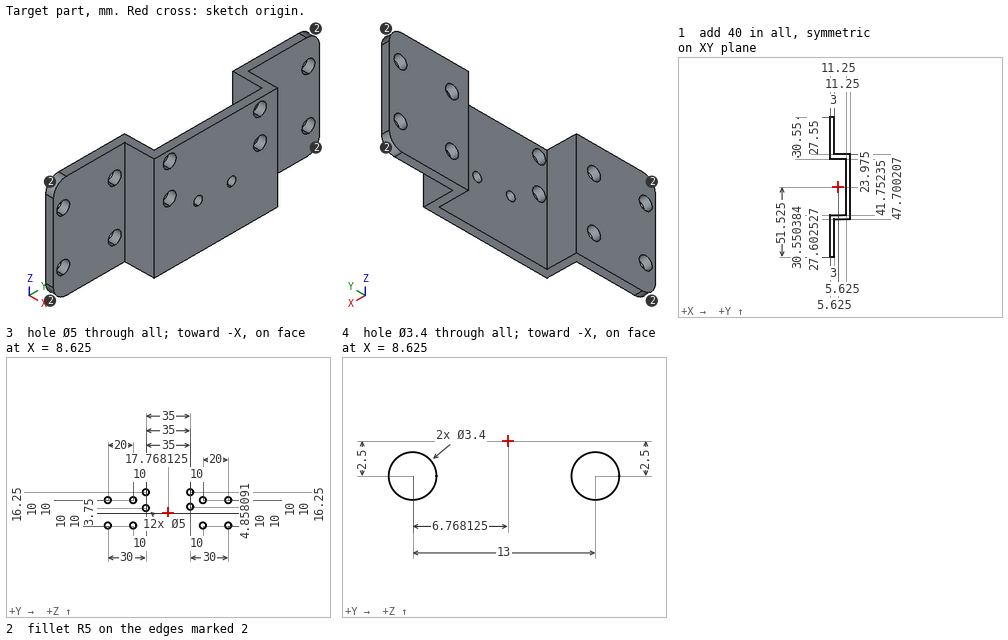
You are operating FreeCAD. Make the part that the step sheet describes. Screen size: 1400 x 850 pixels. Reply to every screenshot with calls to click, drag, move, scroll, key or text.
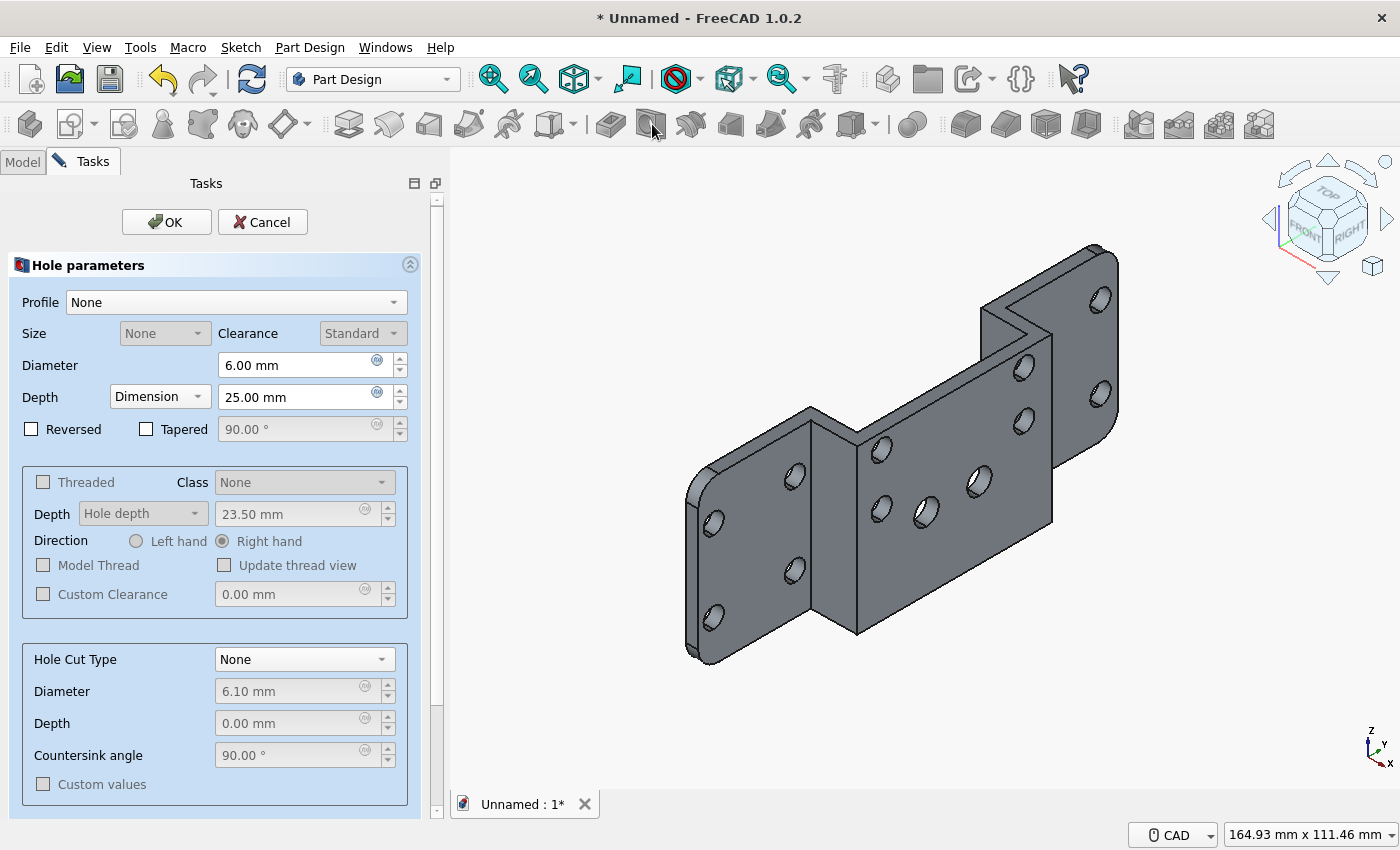
triple_click(305, 365)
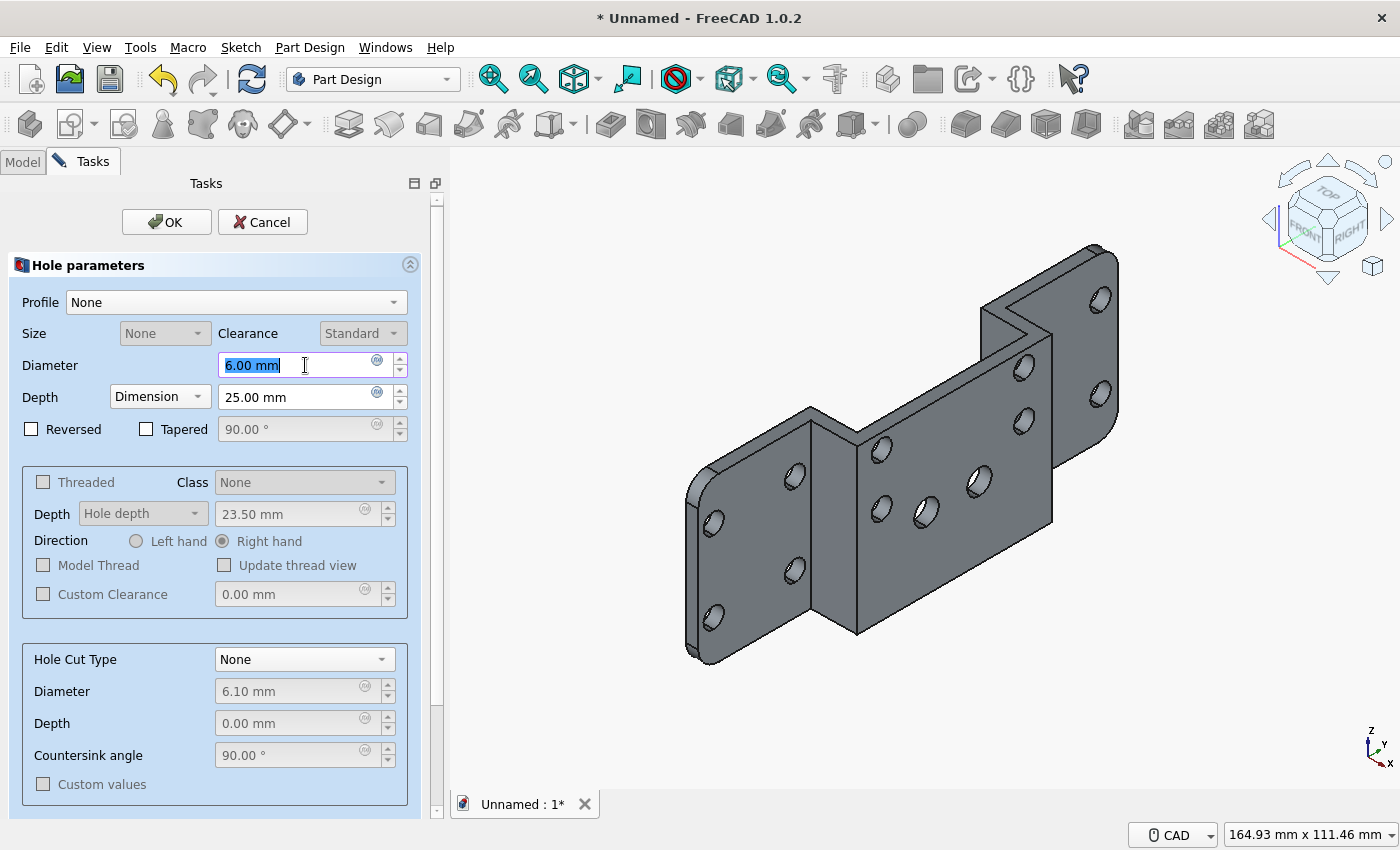
text(3.4)
key(Tab)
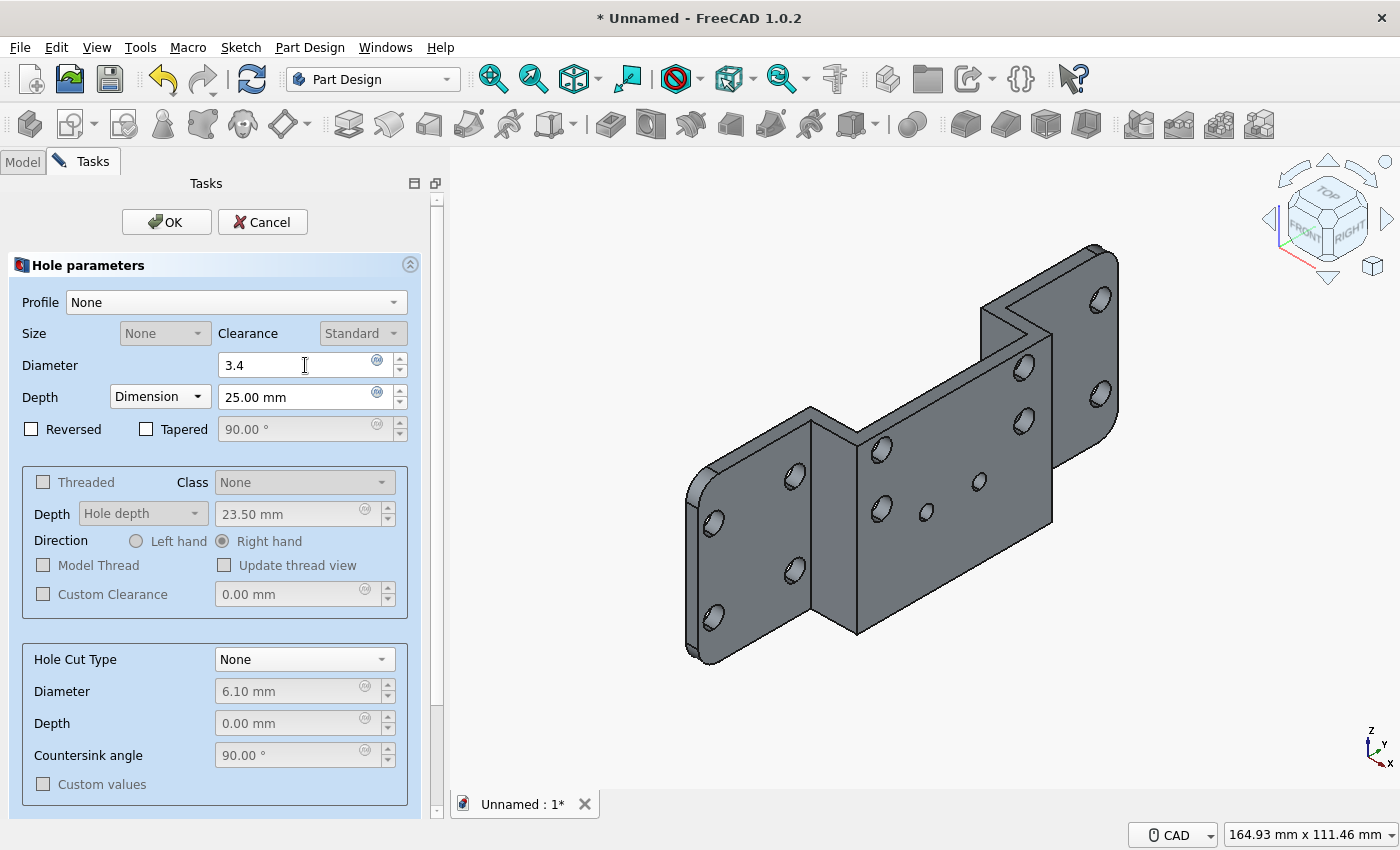
click(161, 396)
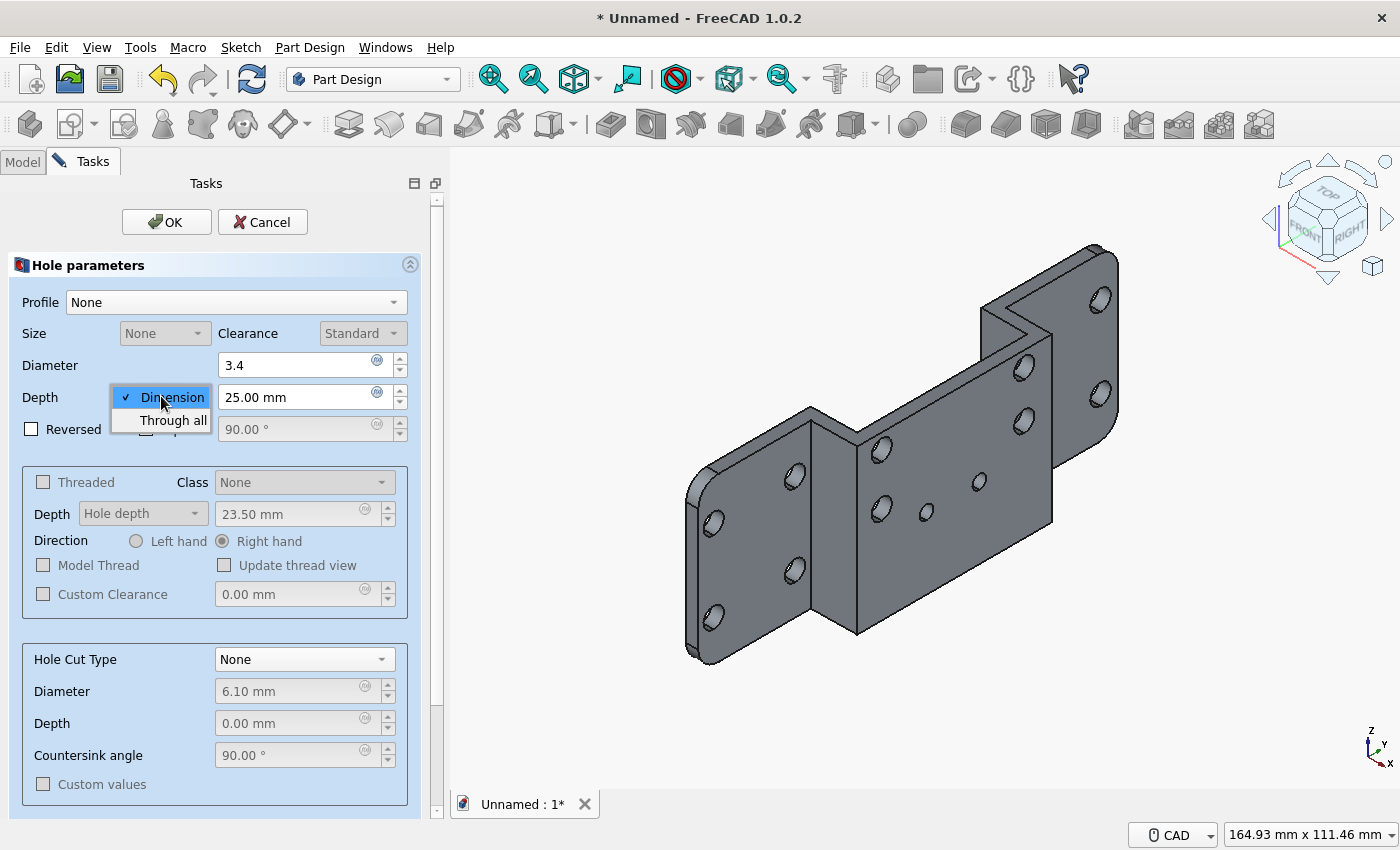
click(160, 420)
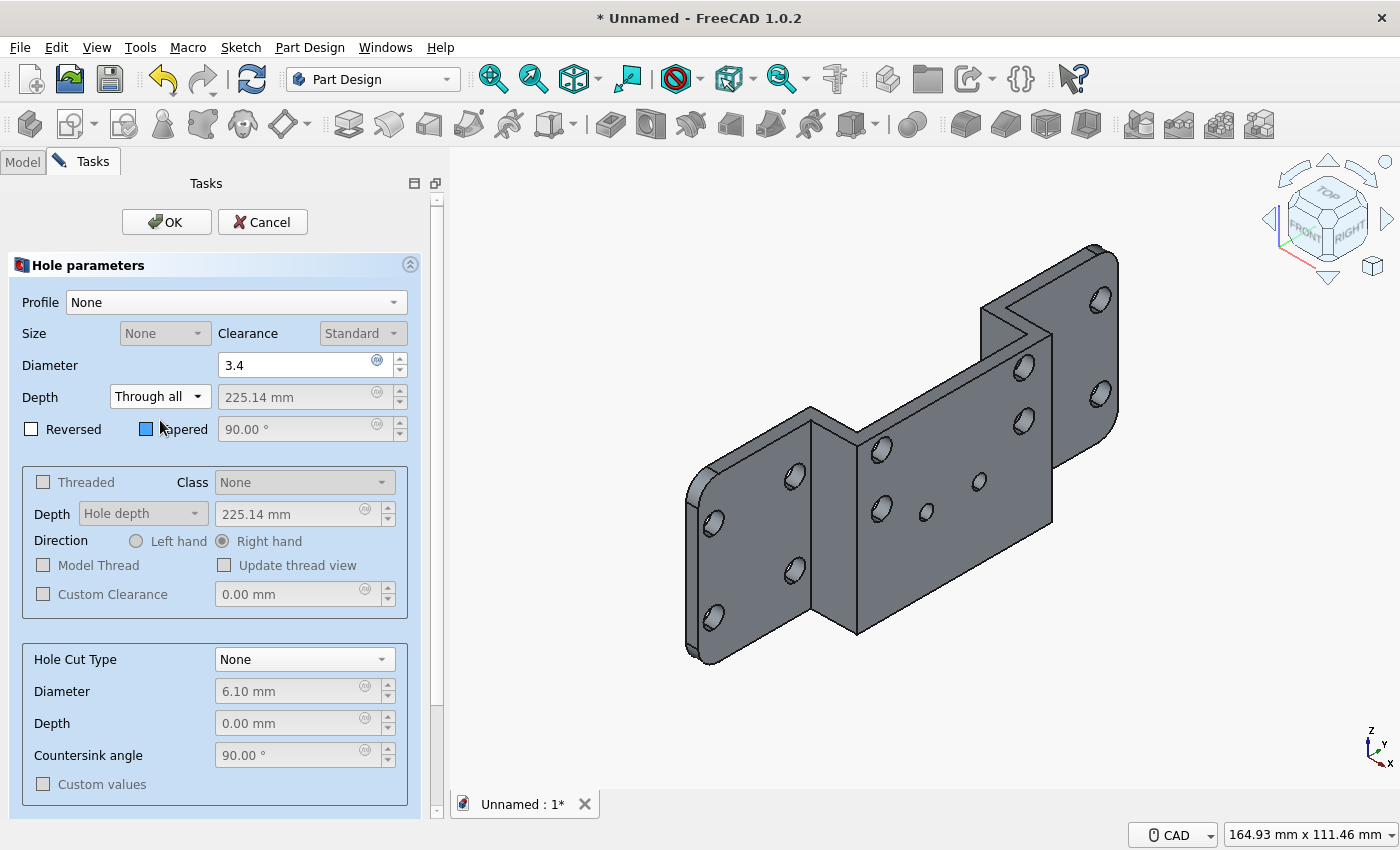
click(167, 222)